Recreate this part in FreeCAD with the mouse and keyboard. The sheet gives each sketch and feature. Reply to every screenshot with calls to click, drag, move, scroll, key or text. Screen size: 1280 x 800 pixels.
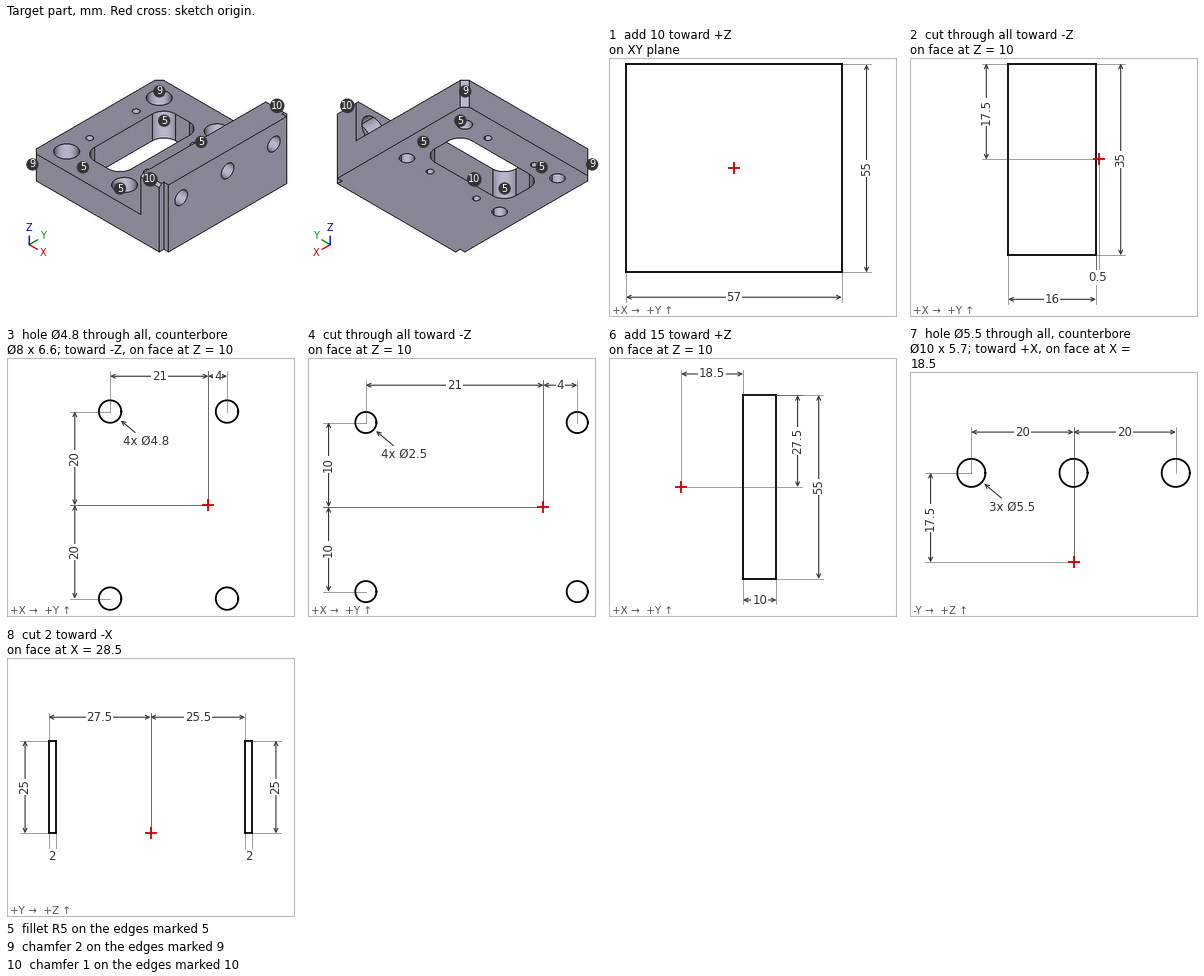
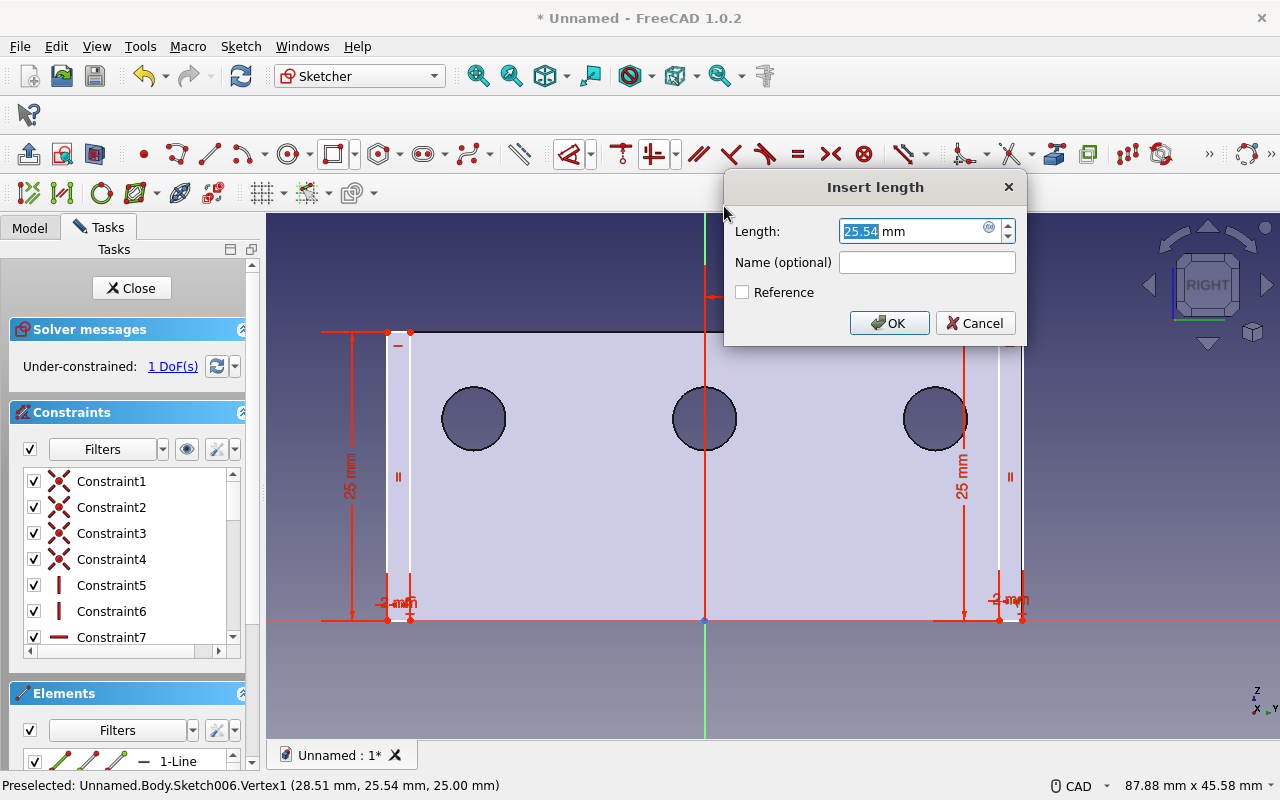
text(25.5)
key(Return)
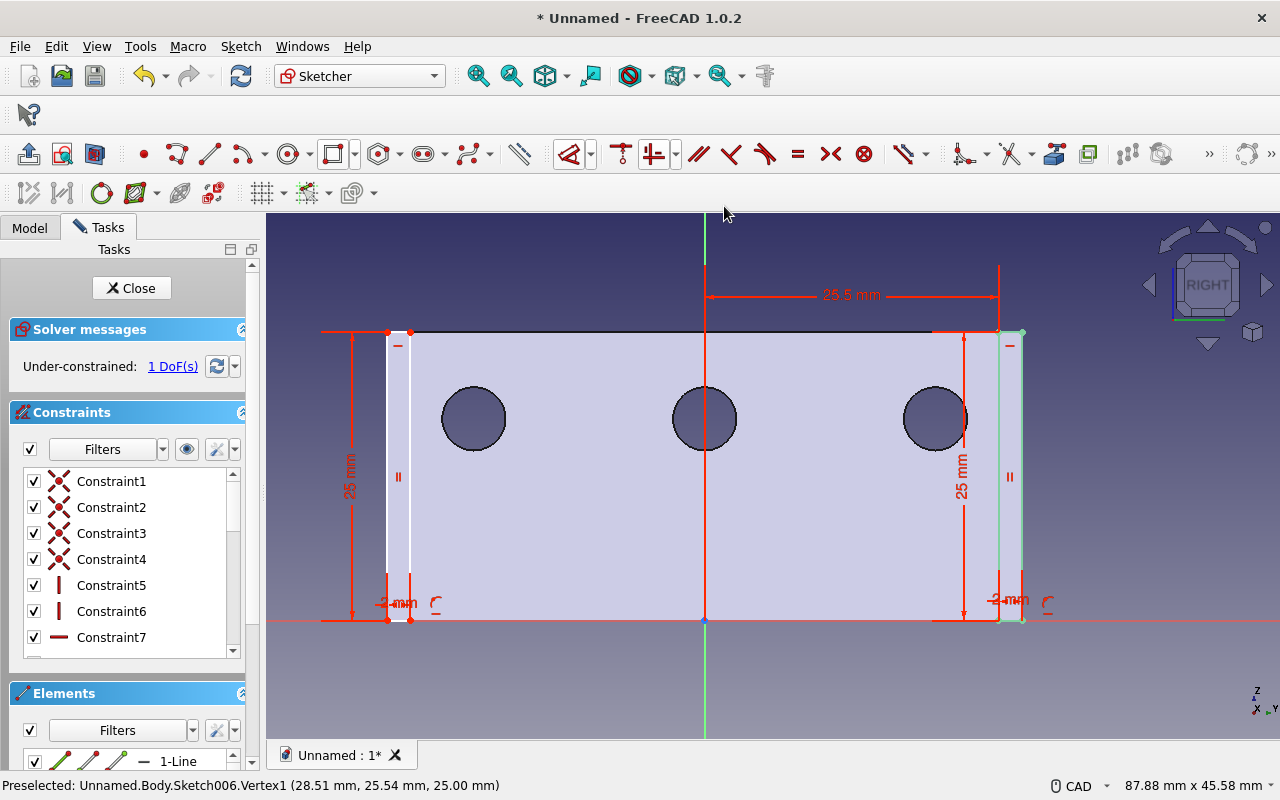
click(387, 332)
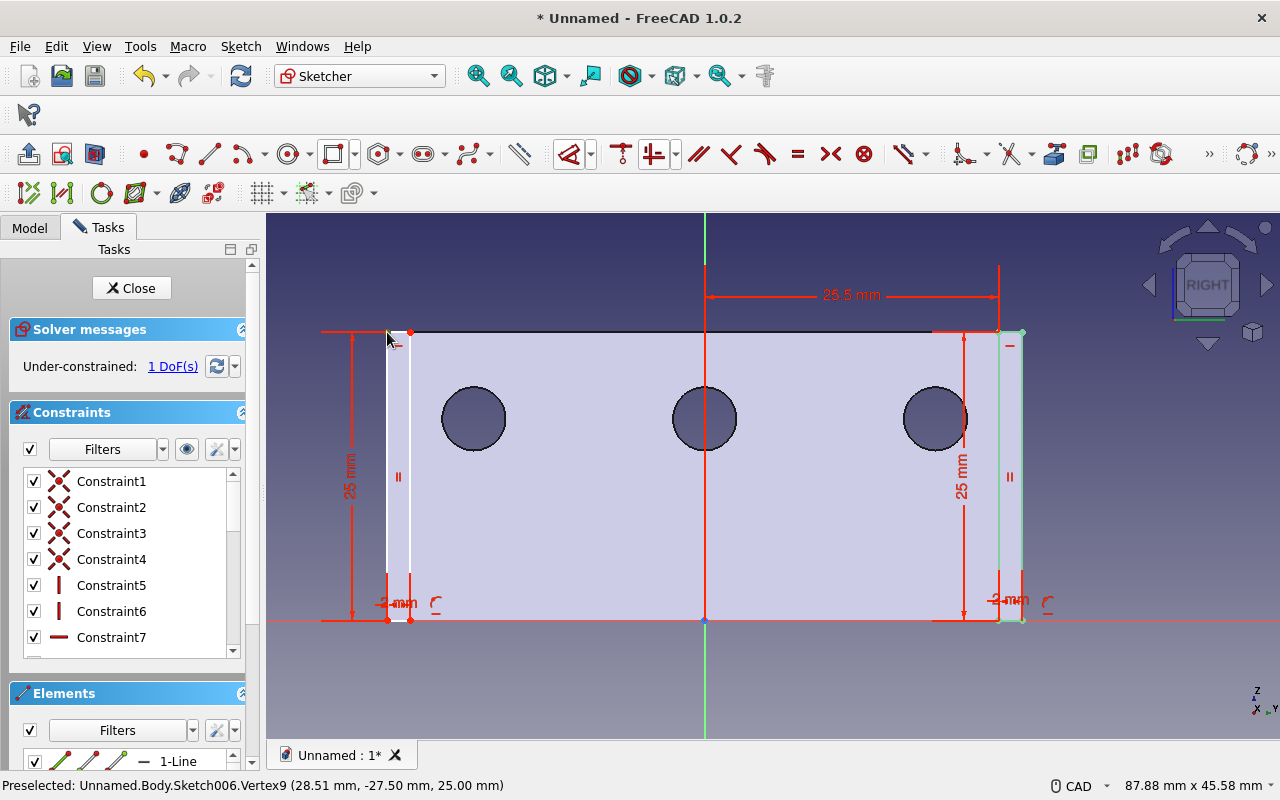
click(590, 154)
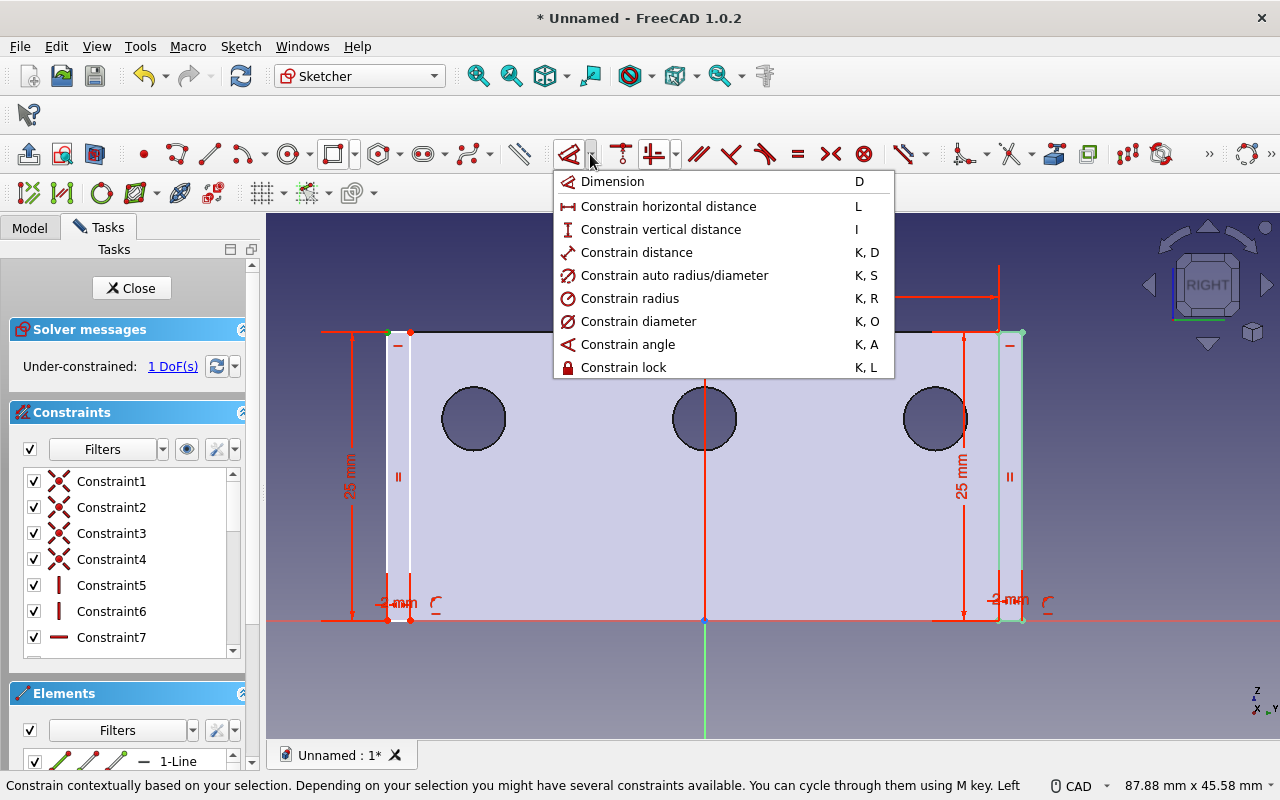
click(724, 206)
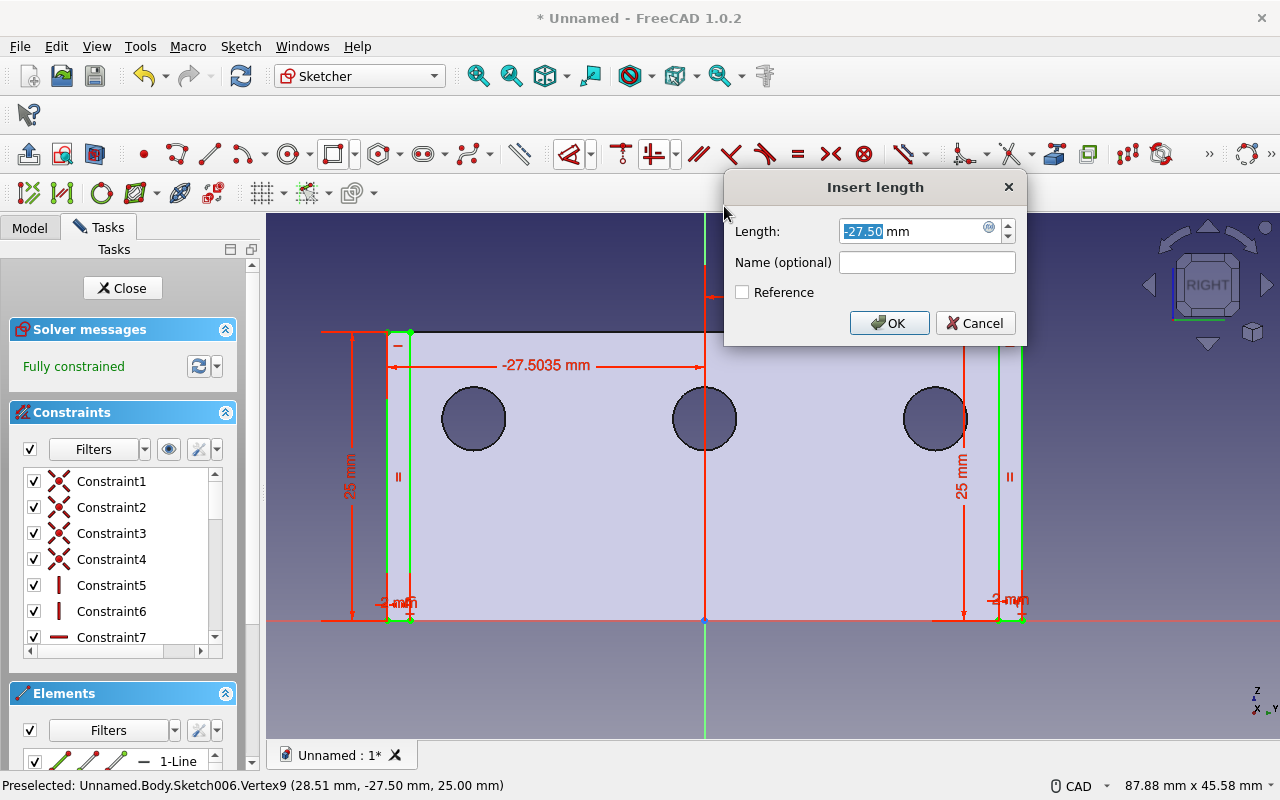
text(-27.5)
key(Return)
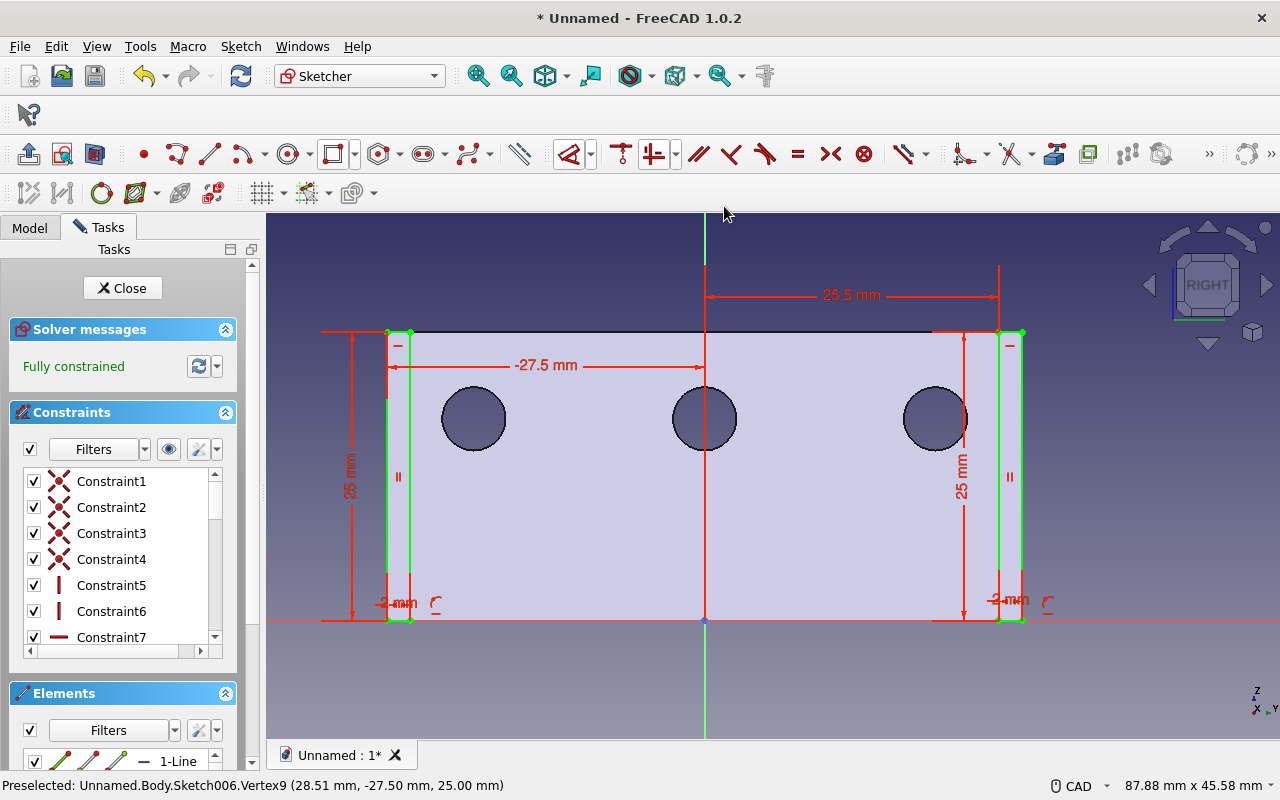
click(123, 288)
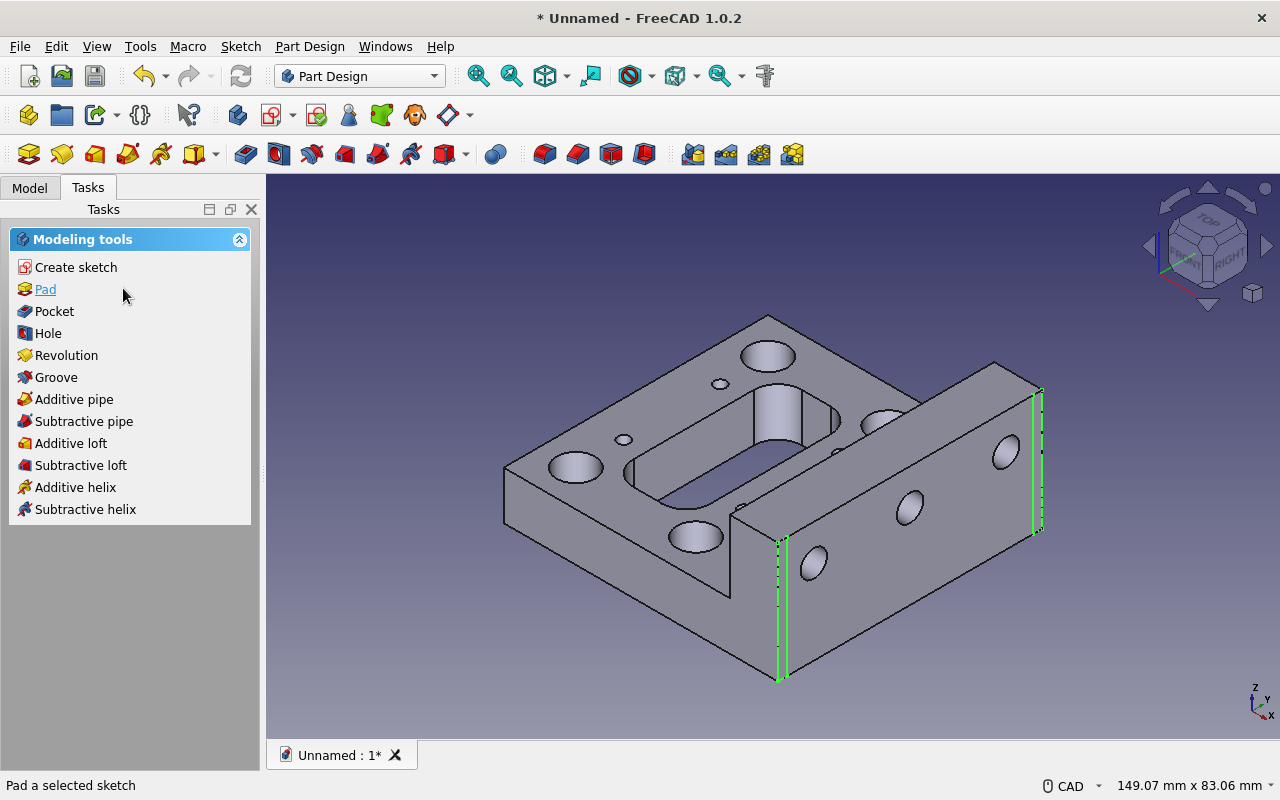
click(246, 154)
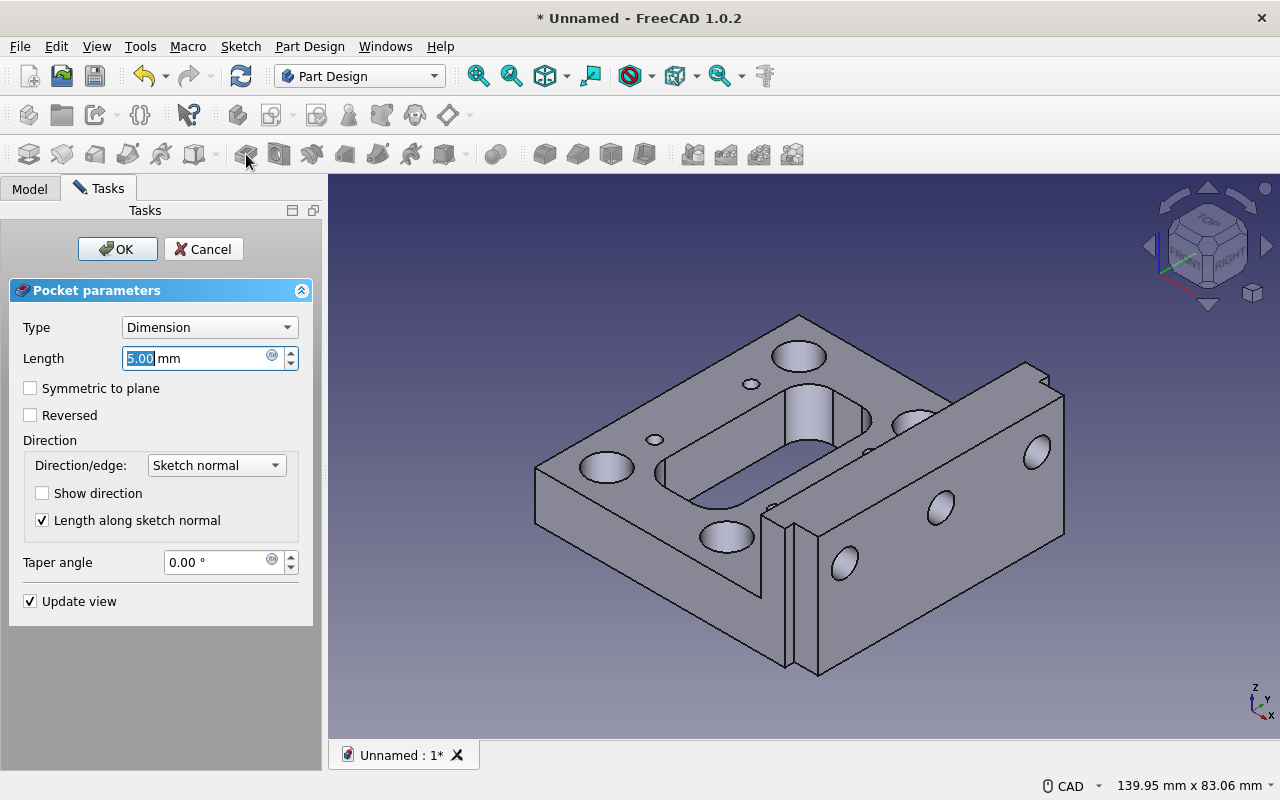
text(2)
key(Tab)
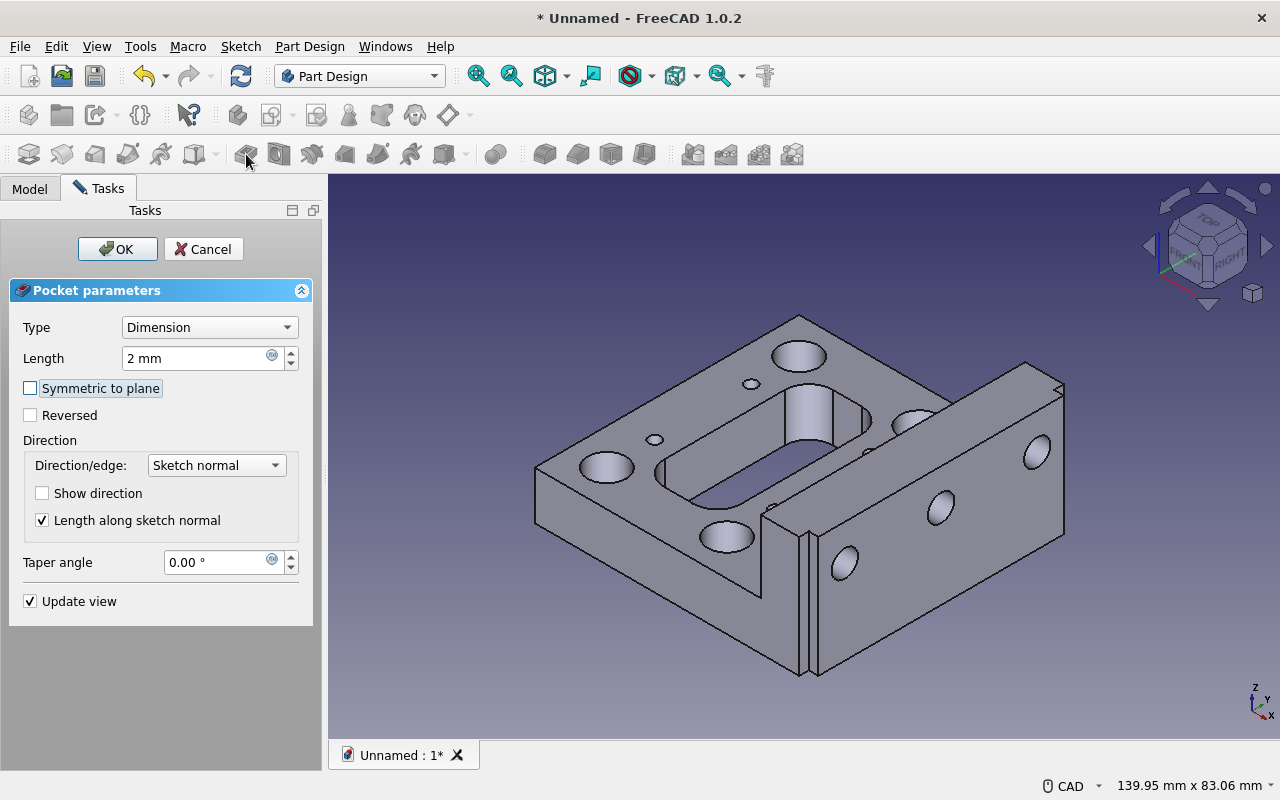
click(118, 249)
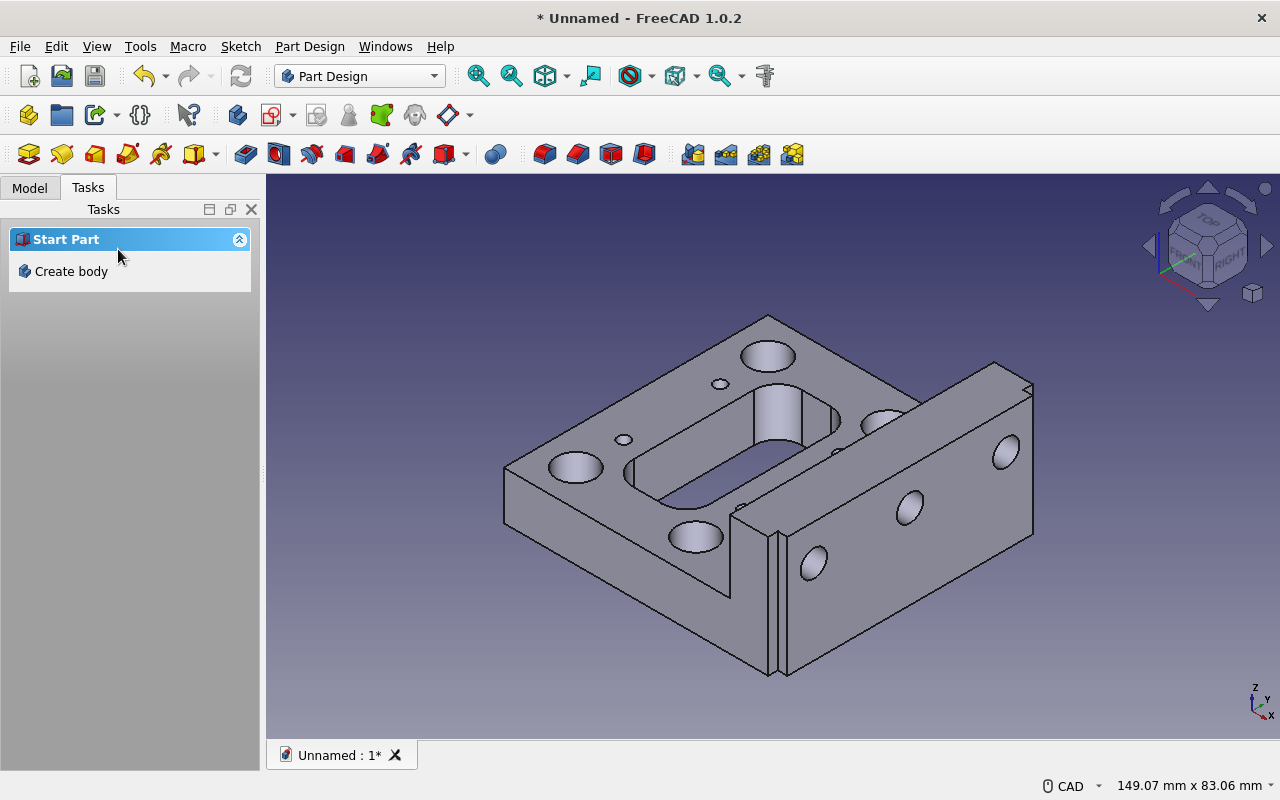
key(2)